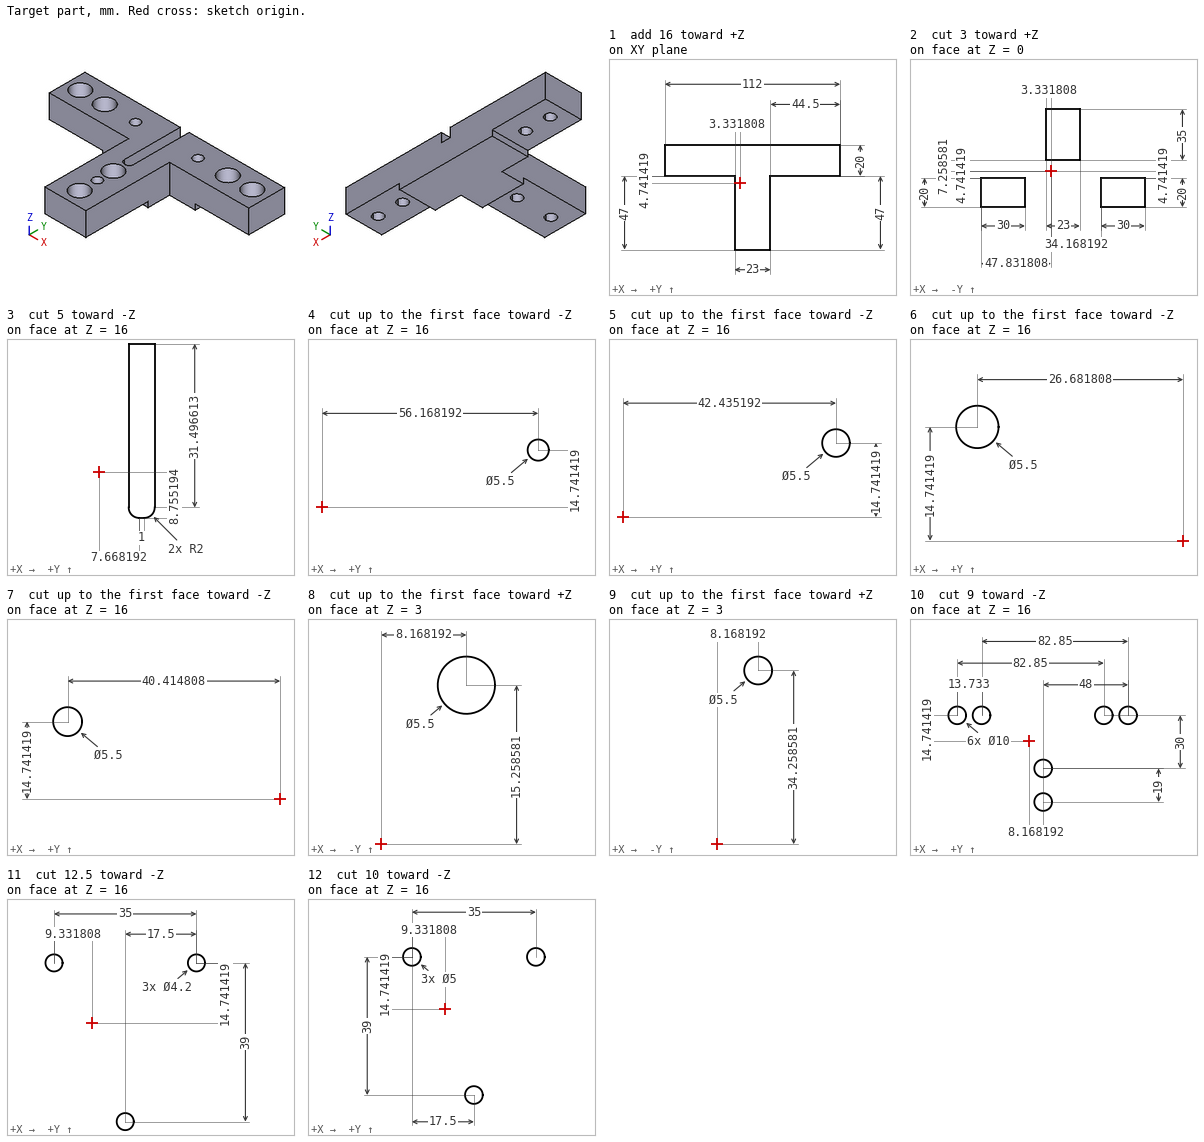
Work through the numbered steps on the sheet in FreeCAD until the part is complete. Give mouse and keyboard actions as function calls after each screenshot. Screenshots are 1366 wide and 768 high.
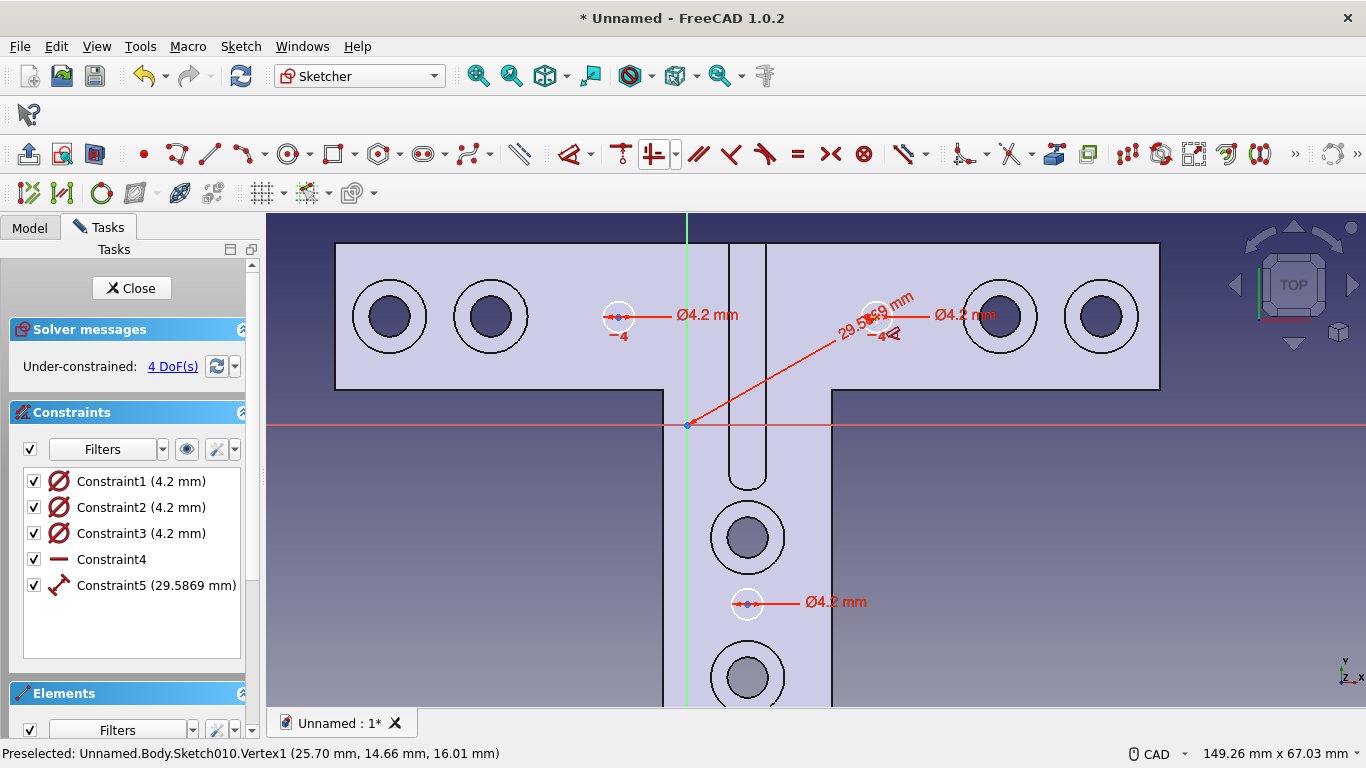
click(619, 317)
click(748, 283)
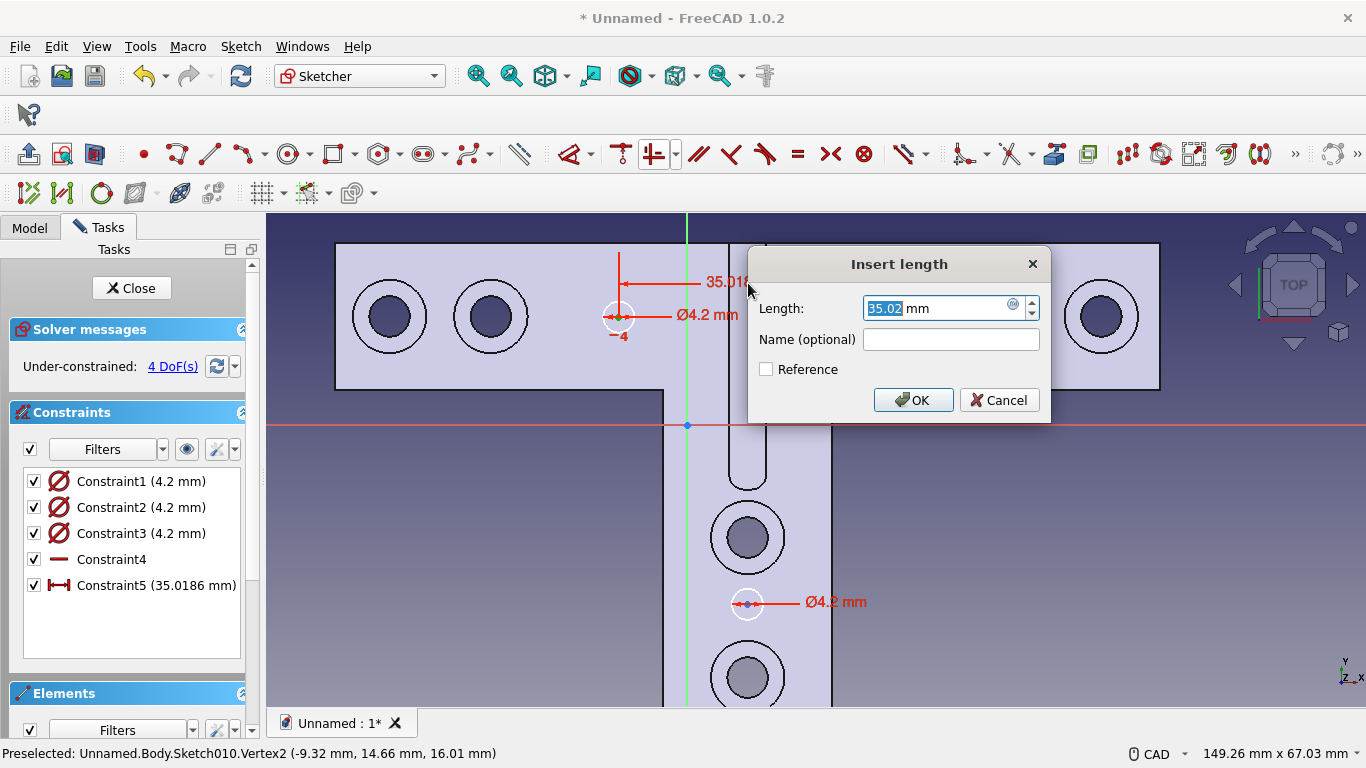
text(35)
key(Return)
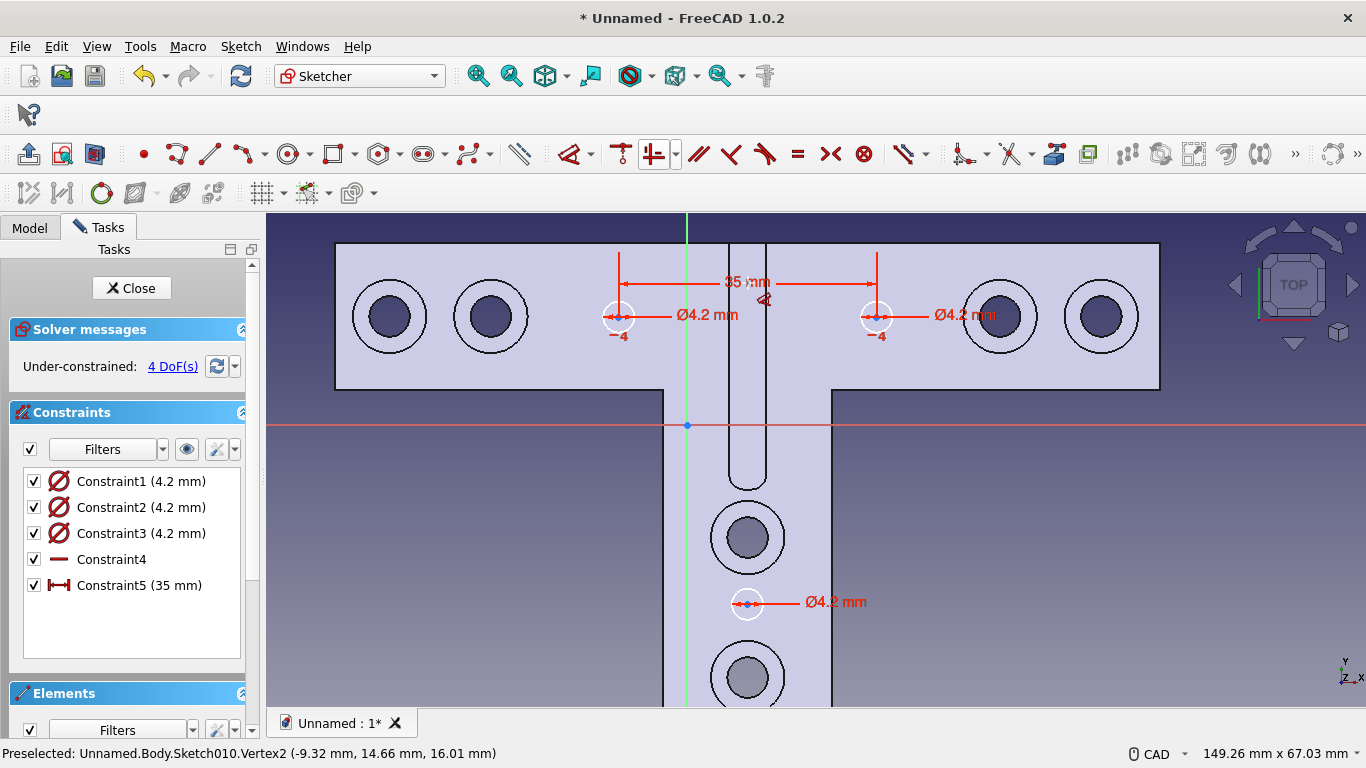
click(877, 317)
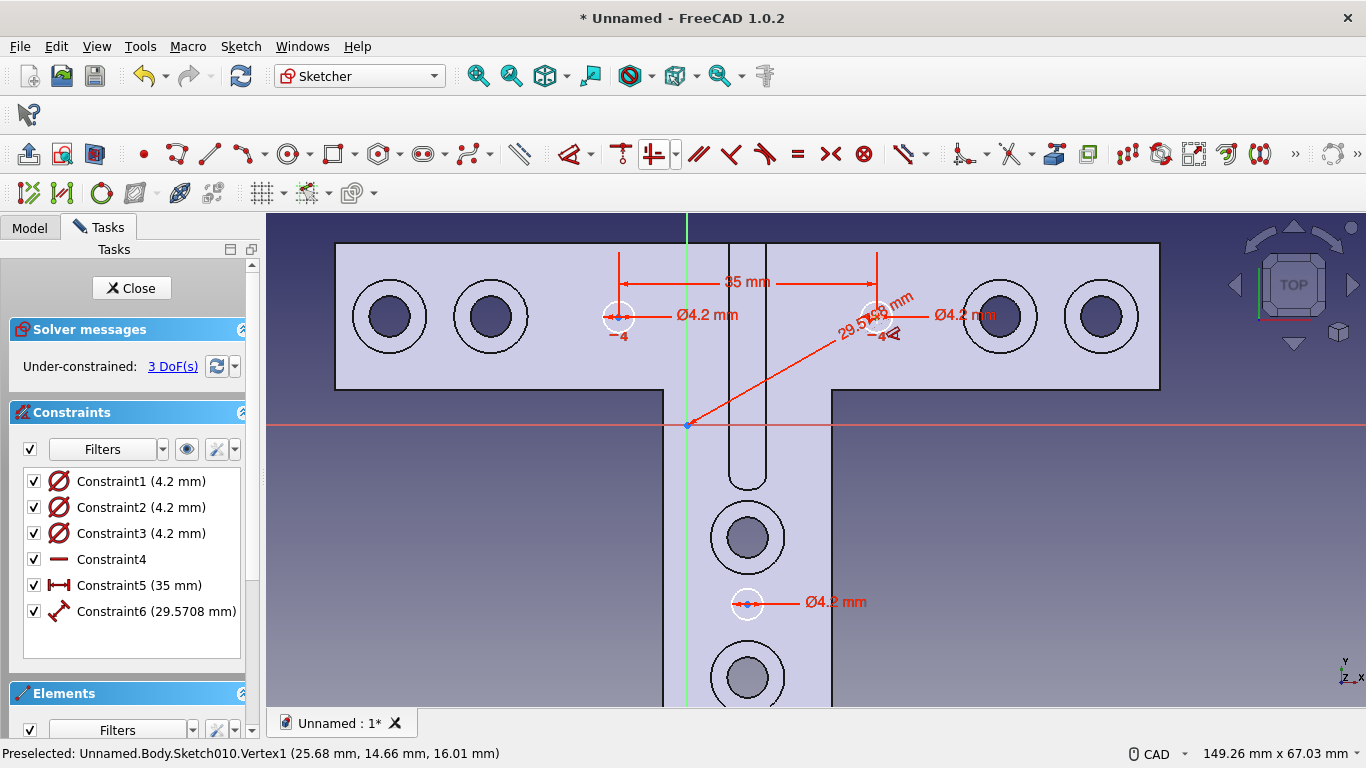
click(747, 604)
click(911, 461)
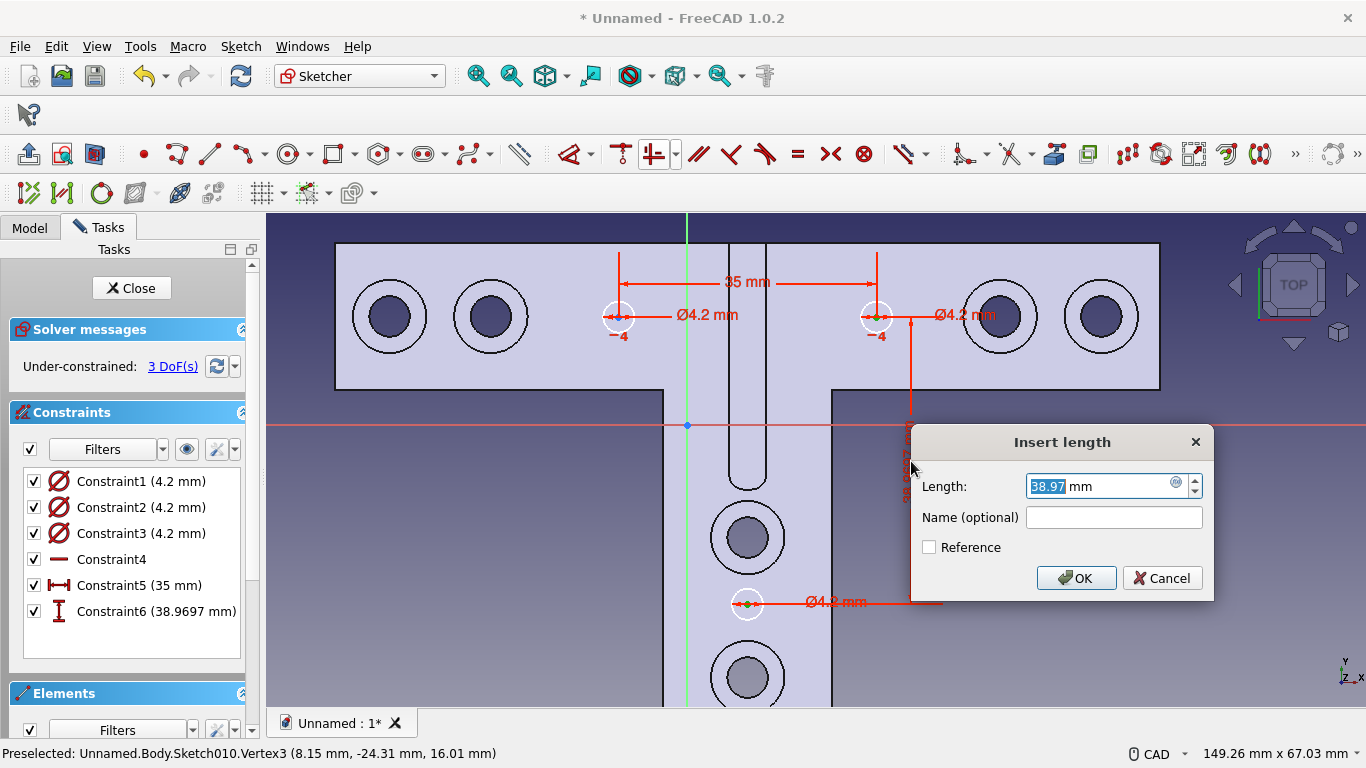
text(39)
key(Return)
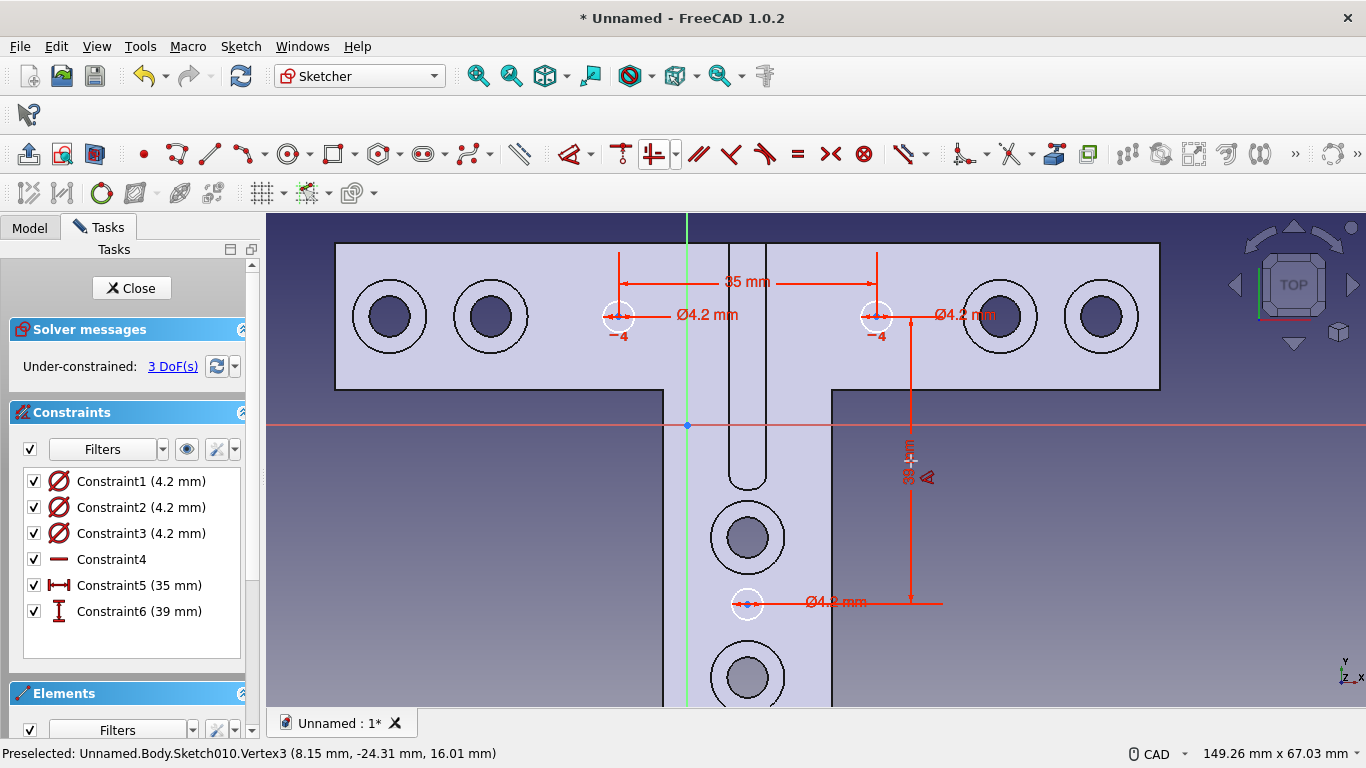
click(877, 317)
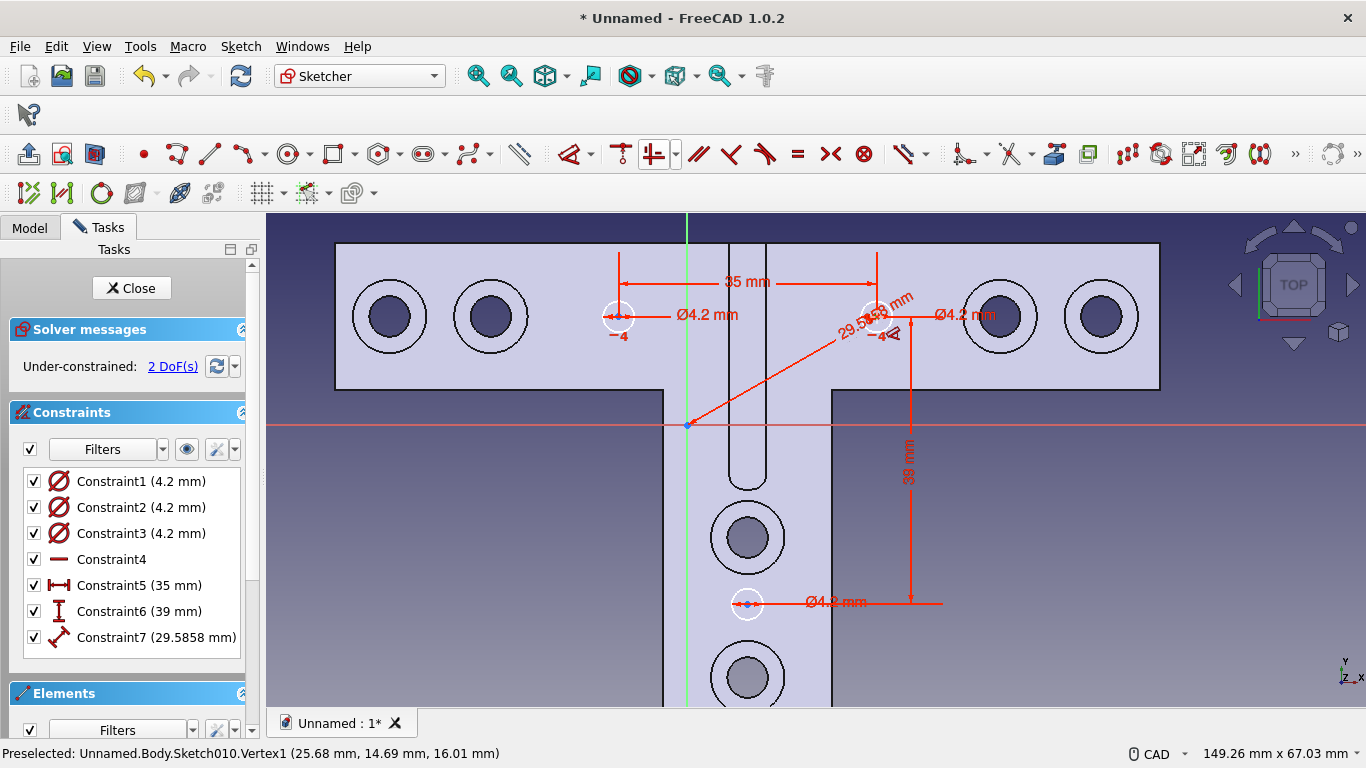
click(747, 604)
click(812, 638)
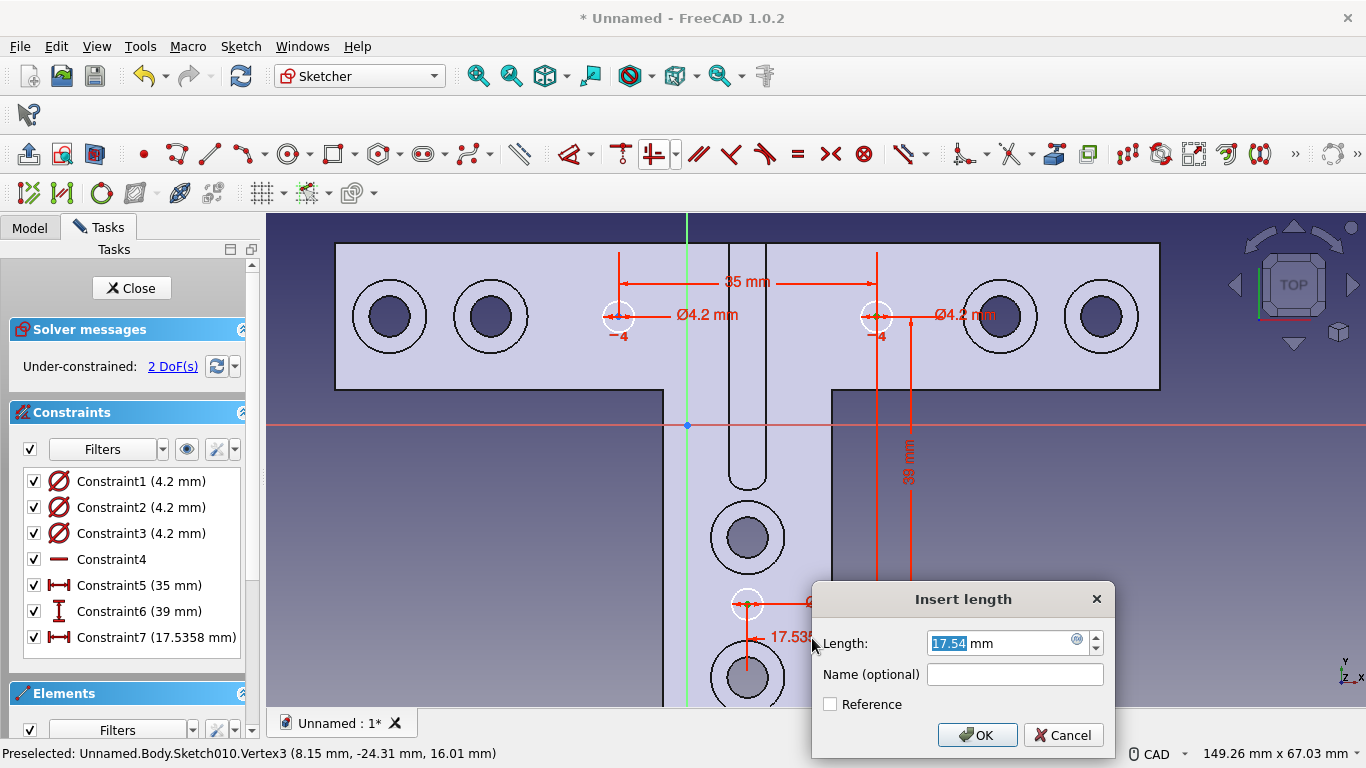
text(17.5)
key(Return)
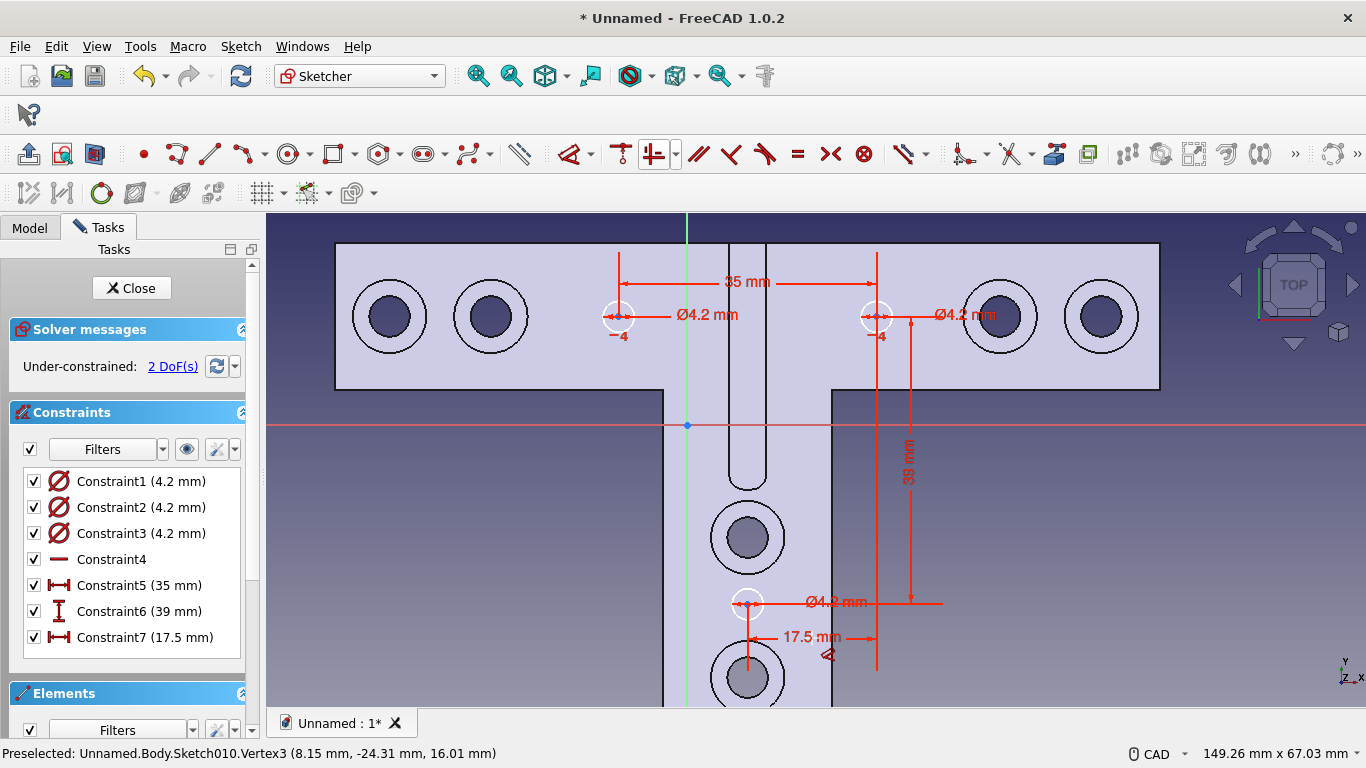
click(619, 317)
click(653, 283)